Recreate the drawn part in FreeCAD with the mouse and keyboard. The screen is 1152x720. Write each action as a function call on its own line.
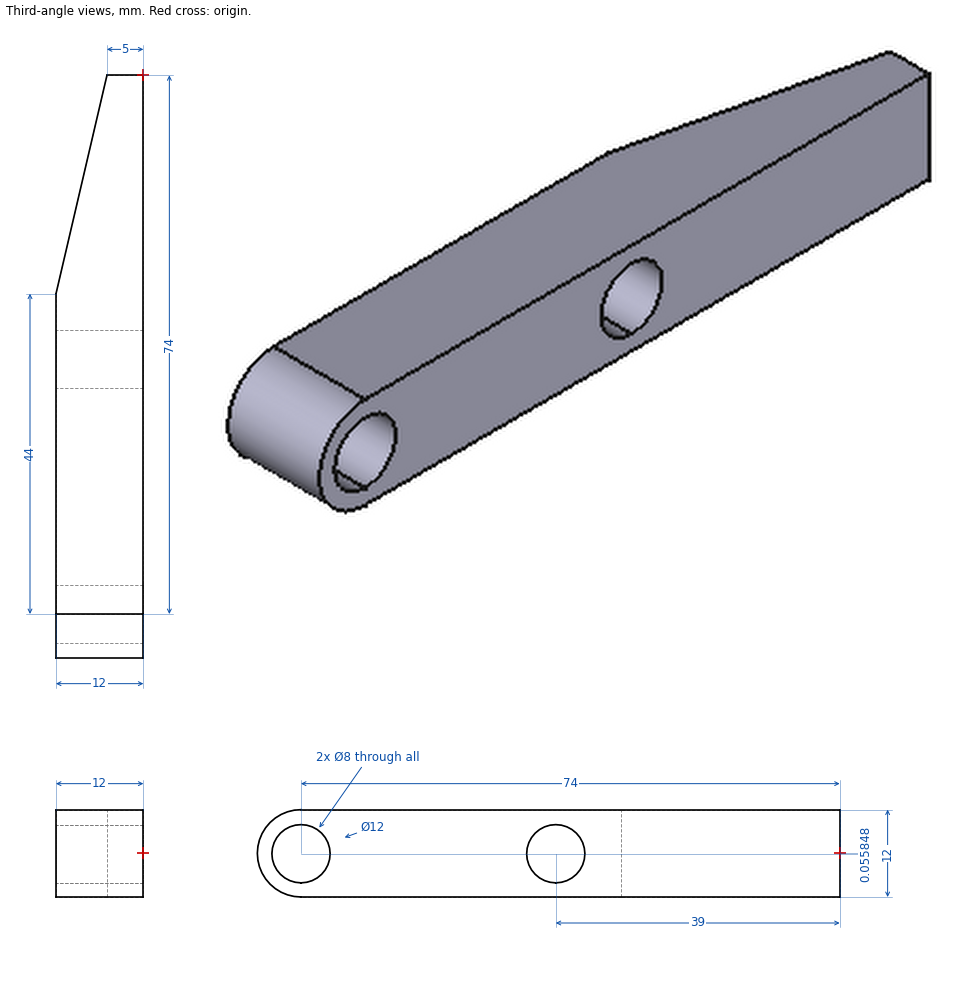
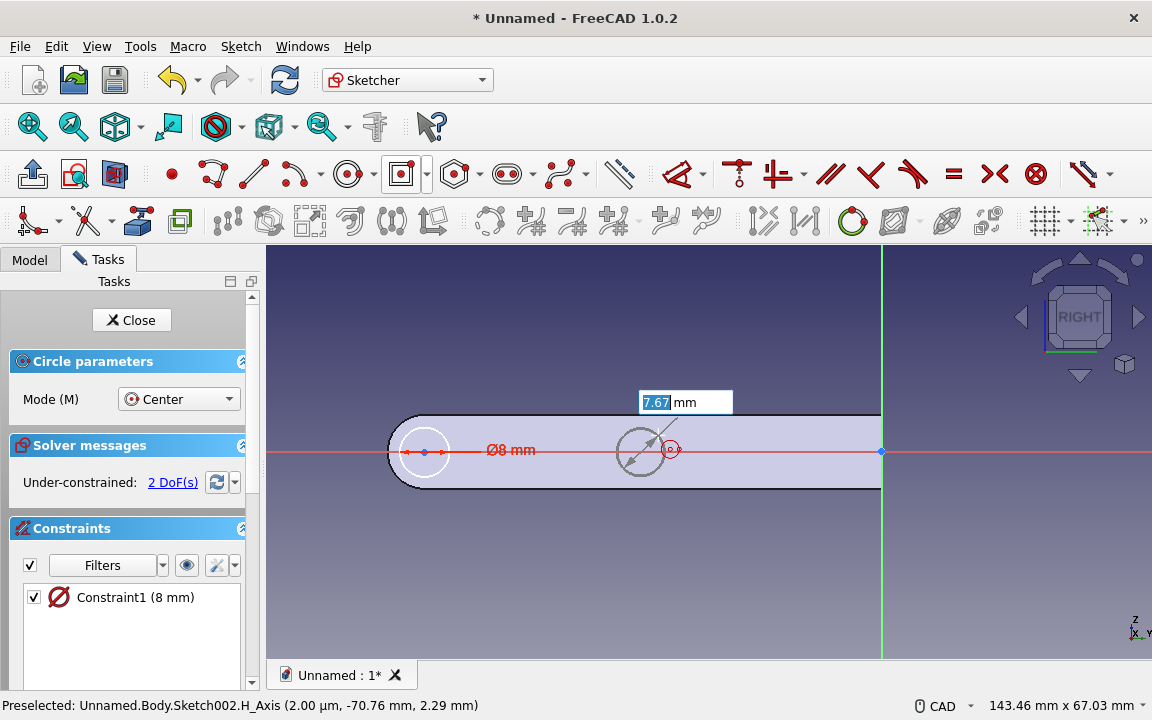
text(8)
key(Return)
key(Escape)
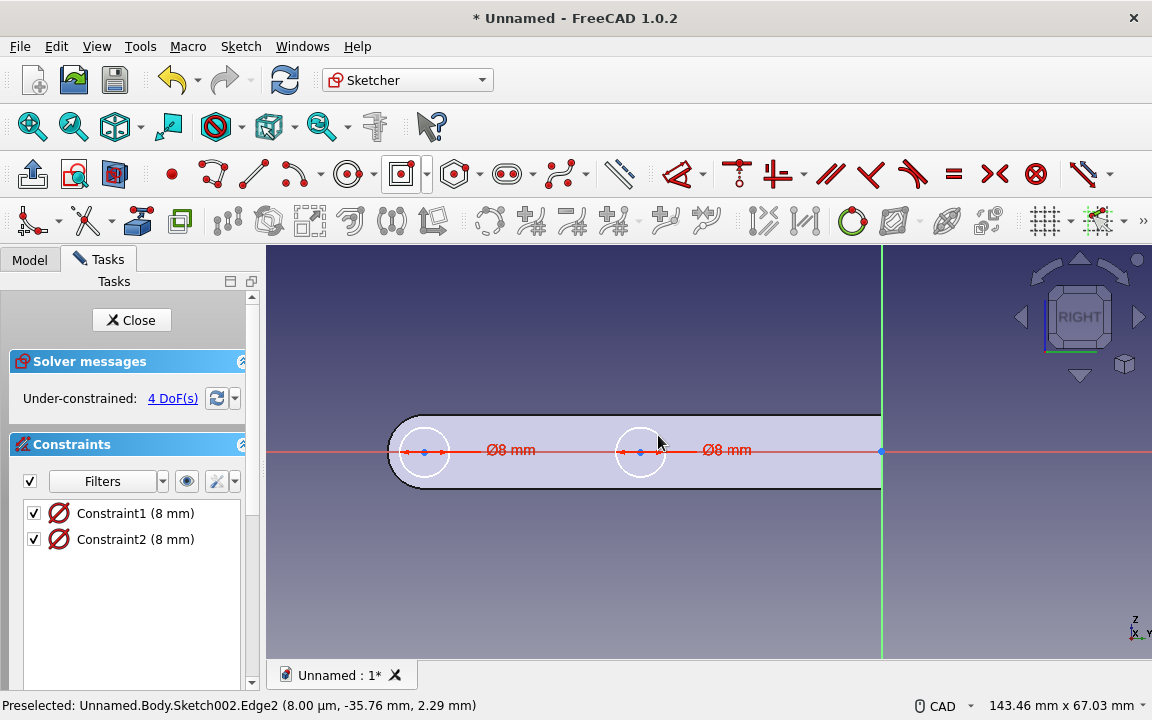
click(425, 452)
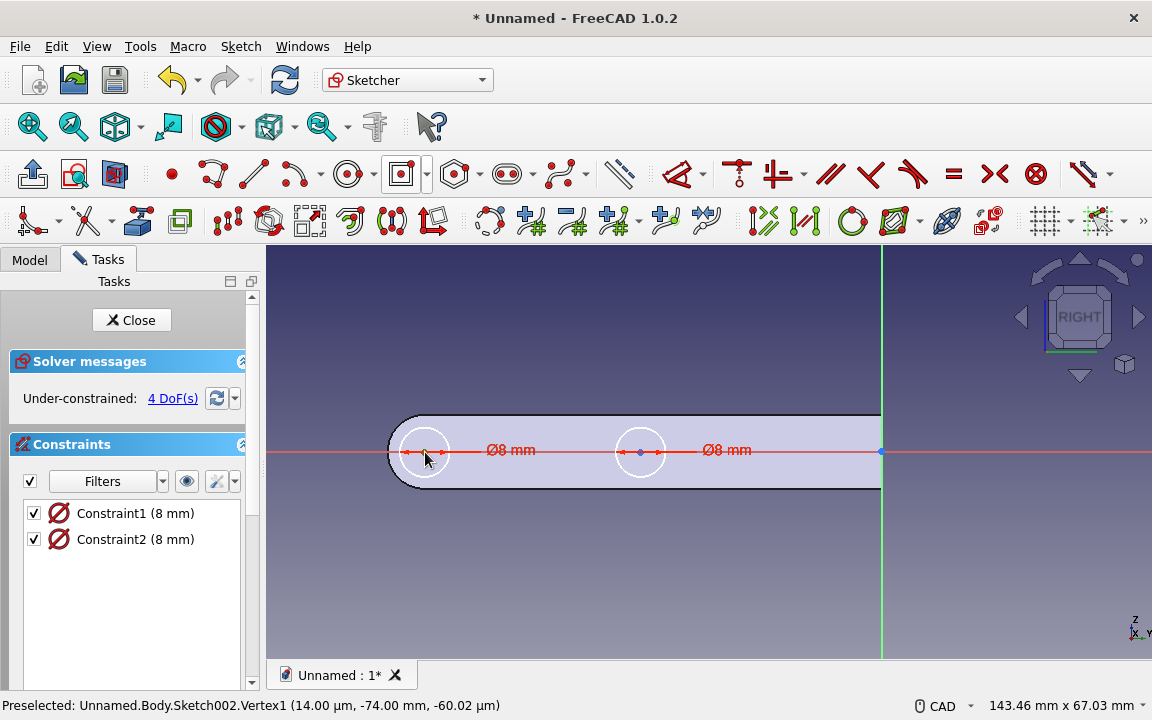
click(641, 452)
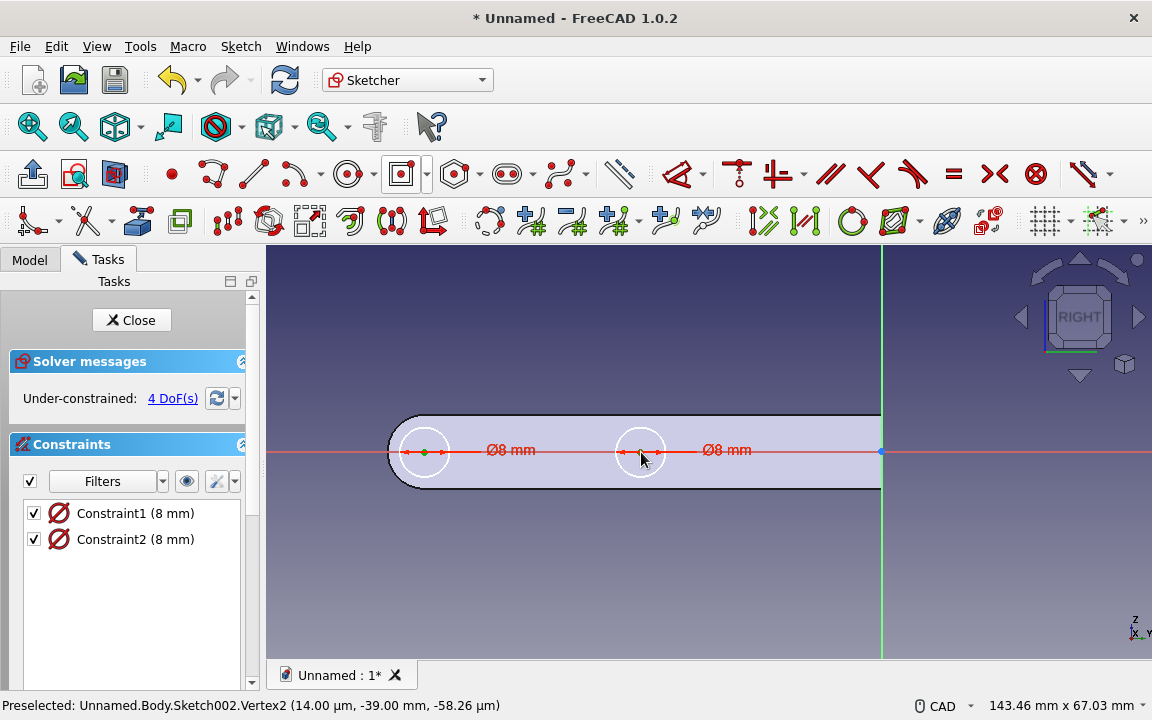
key(h)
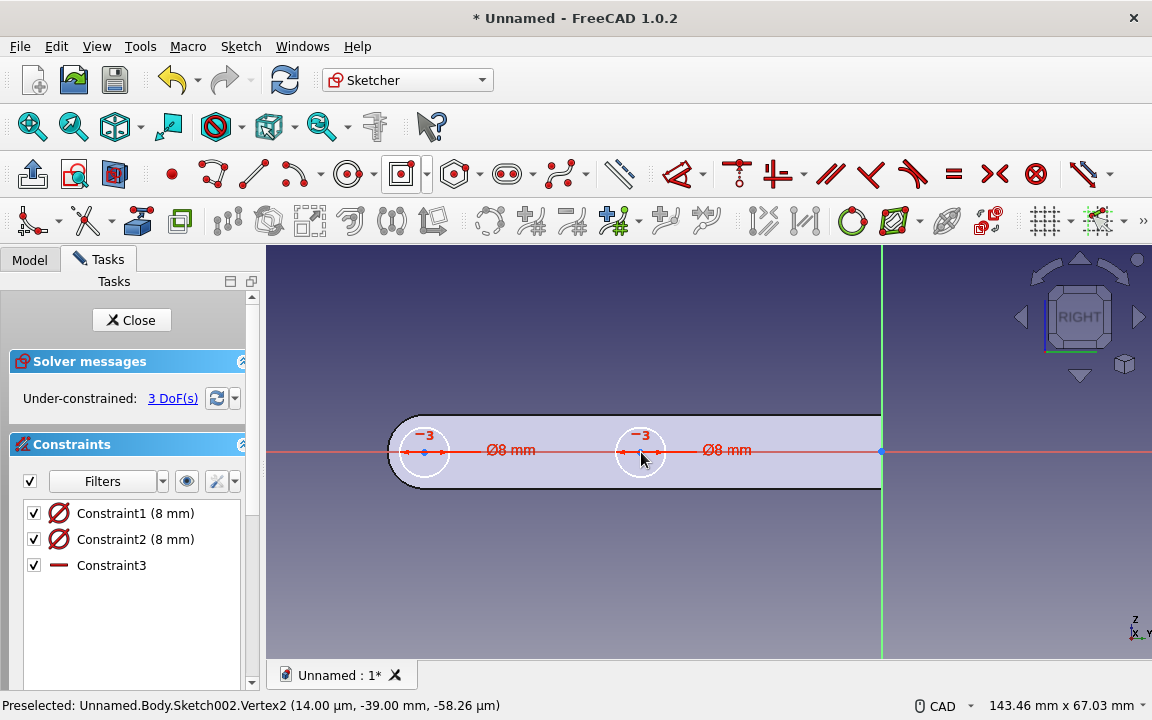
click(425, 452)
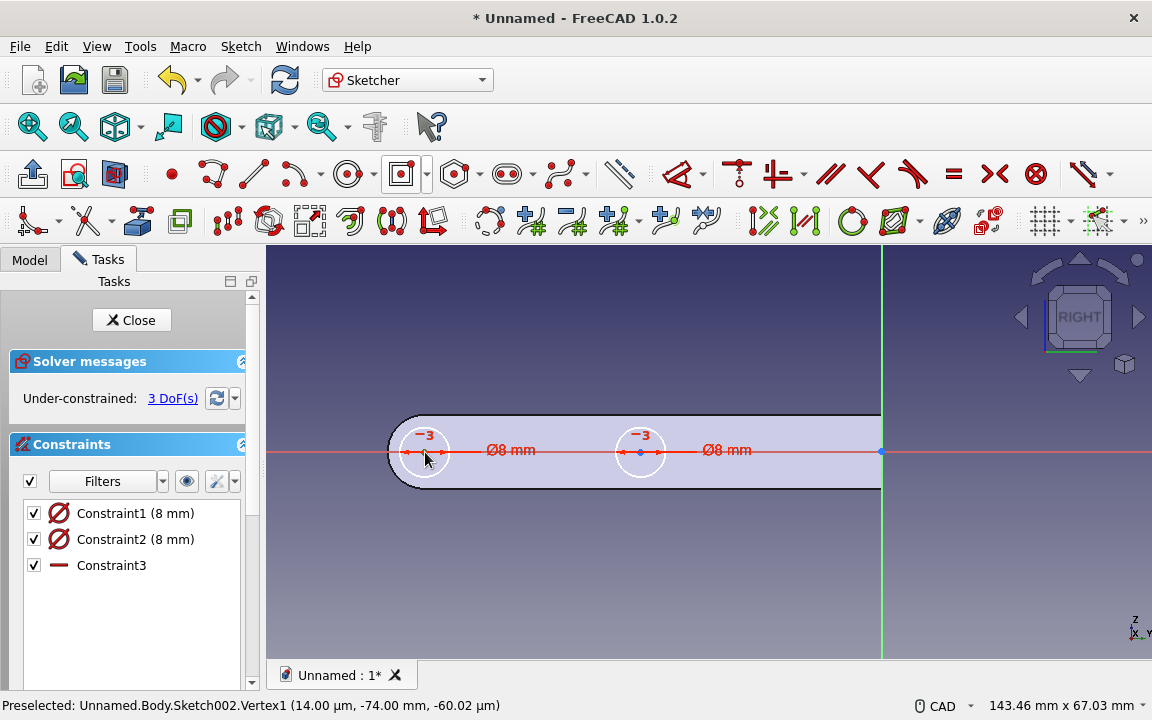
key(l)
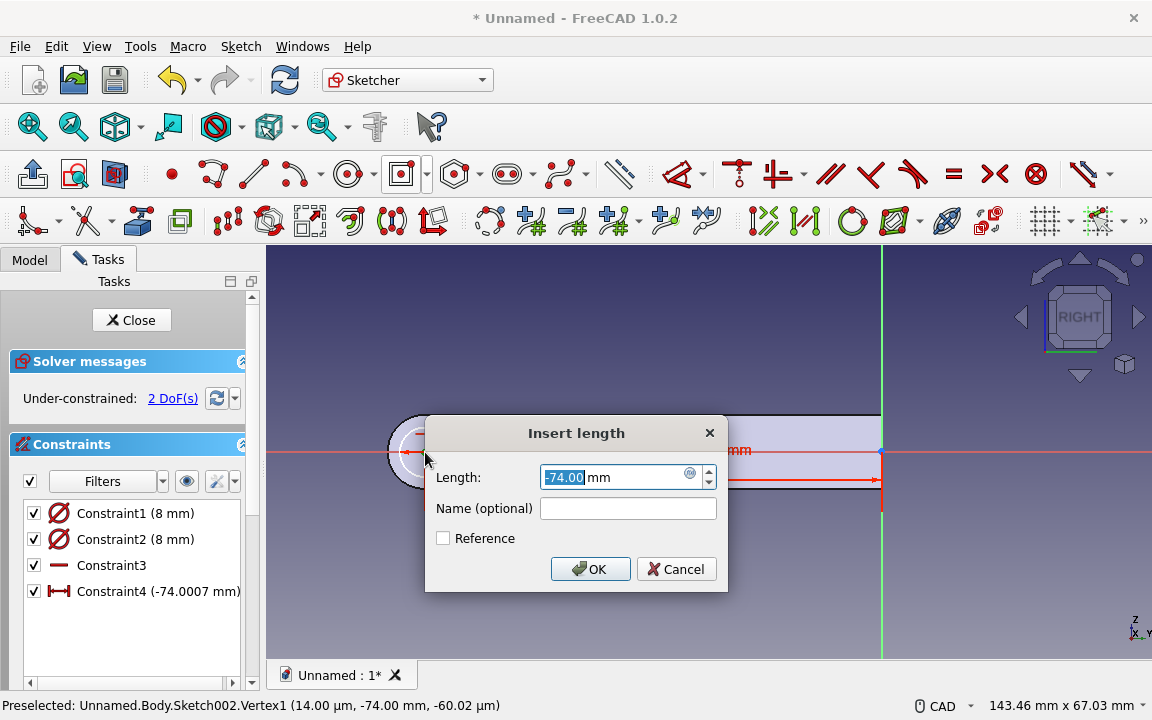
text(-74)
key(Return)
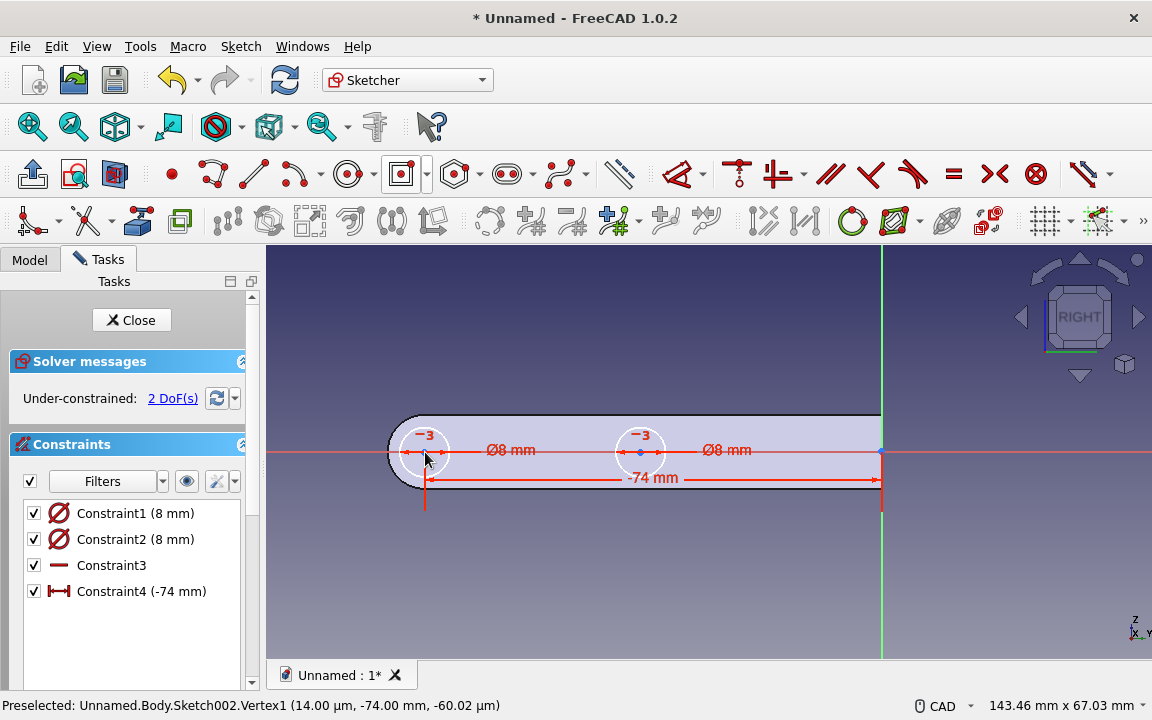
click(641, 452)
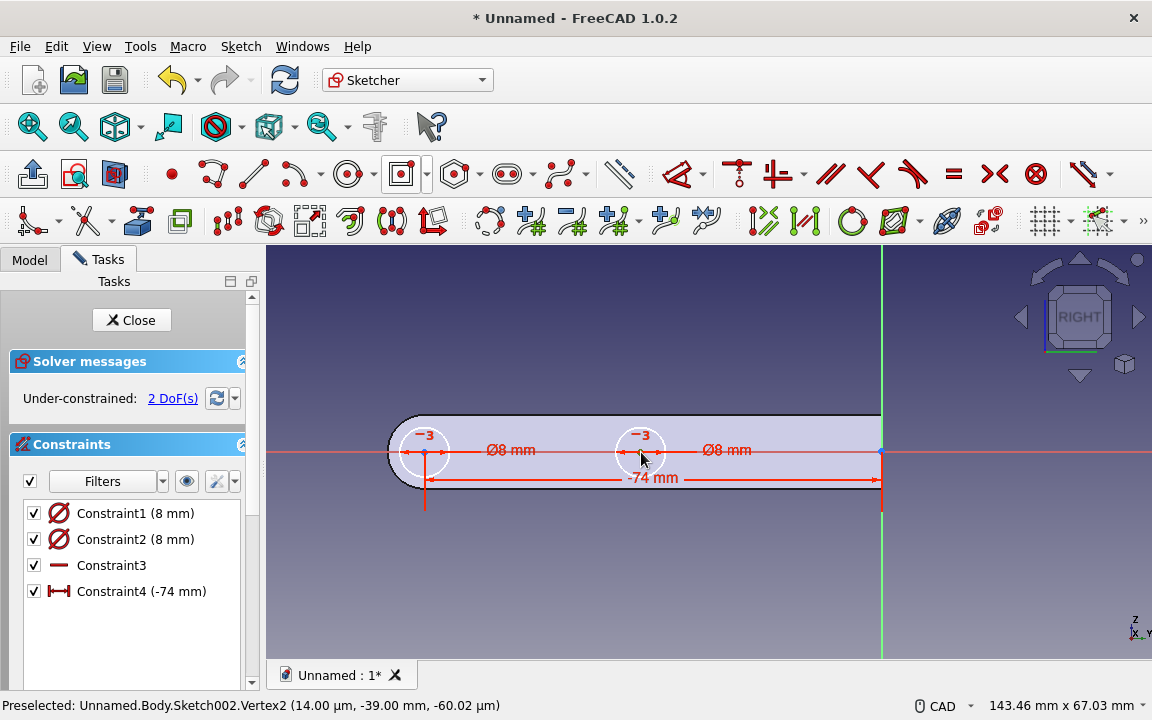
key(l)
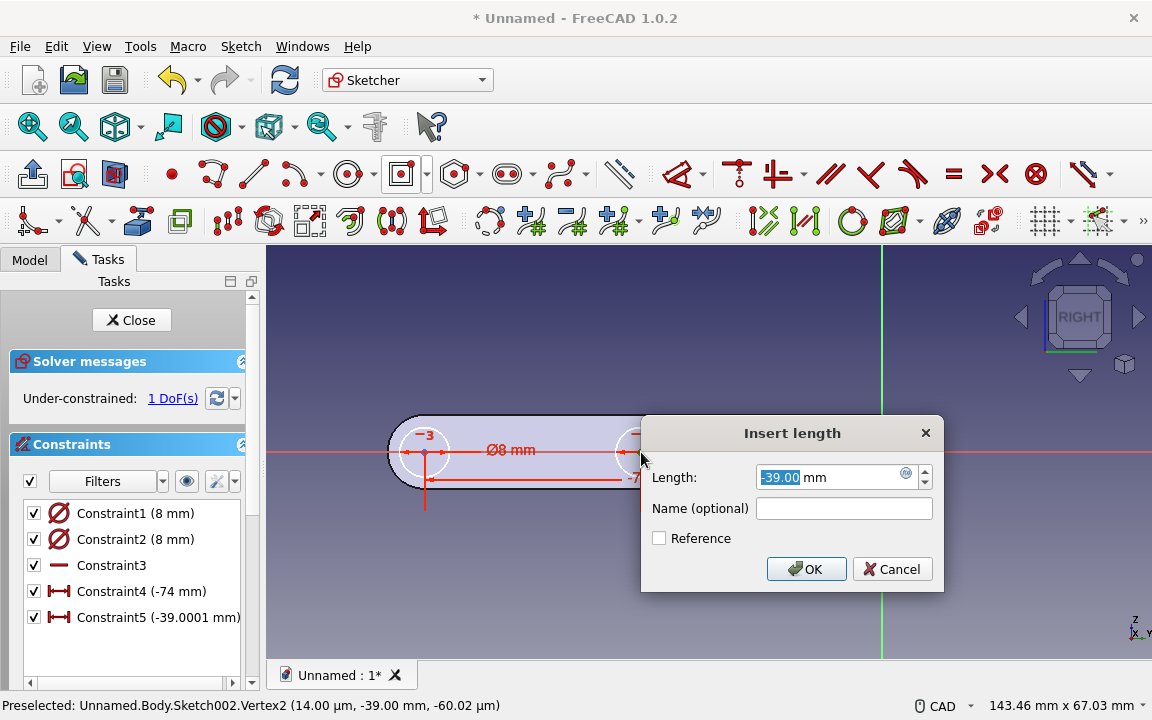
text(-39)
key(Return)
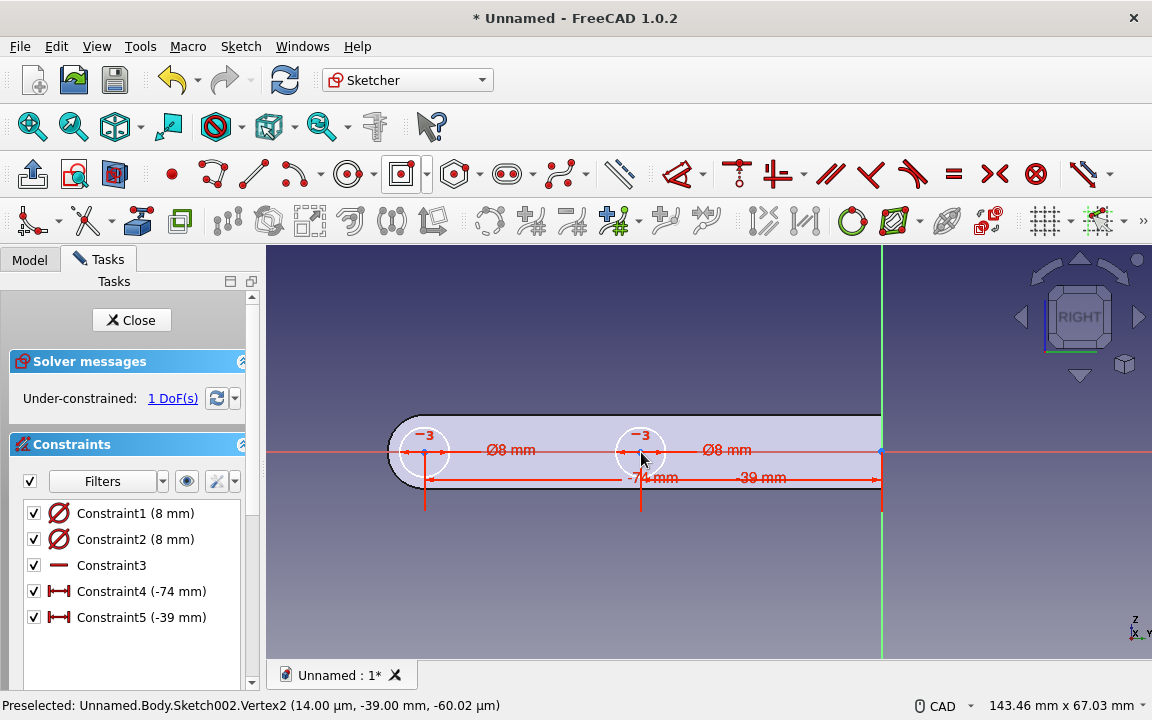
scroll(425, 452, up, 24)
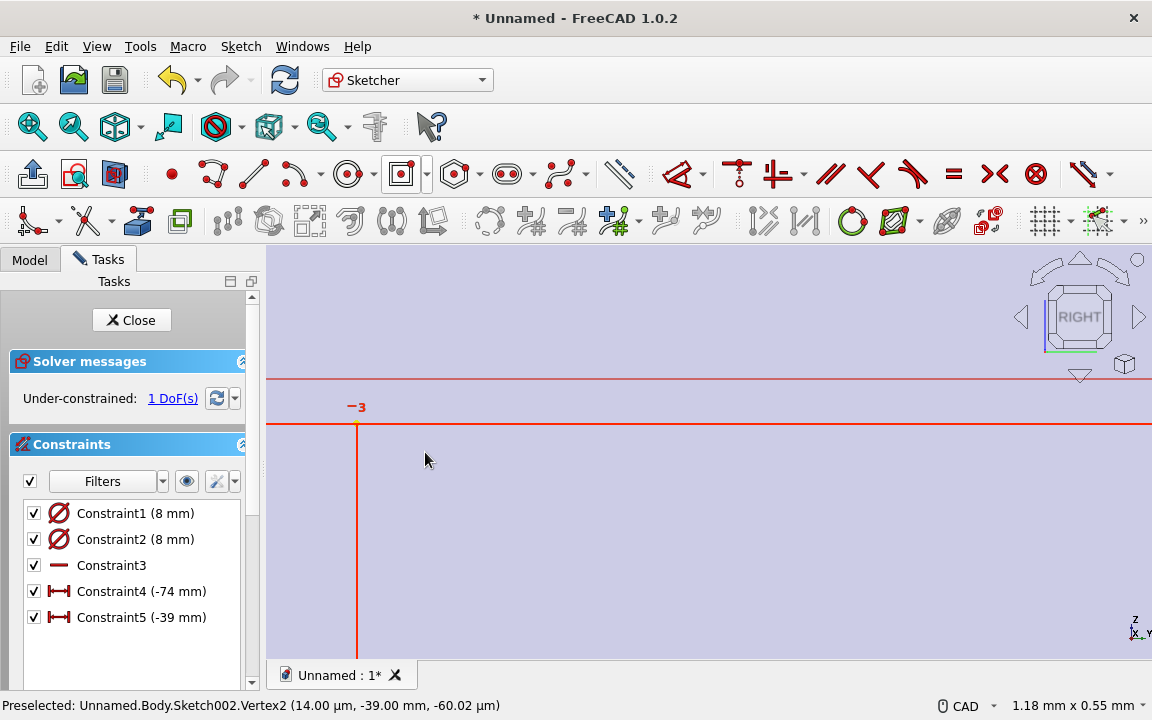
click(357, 424)